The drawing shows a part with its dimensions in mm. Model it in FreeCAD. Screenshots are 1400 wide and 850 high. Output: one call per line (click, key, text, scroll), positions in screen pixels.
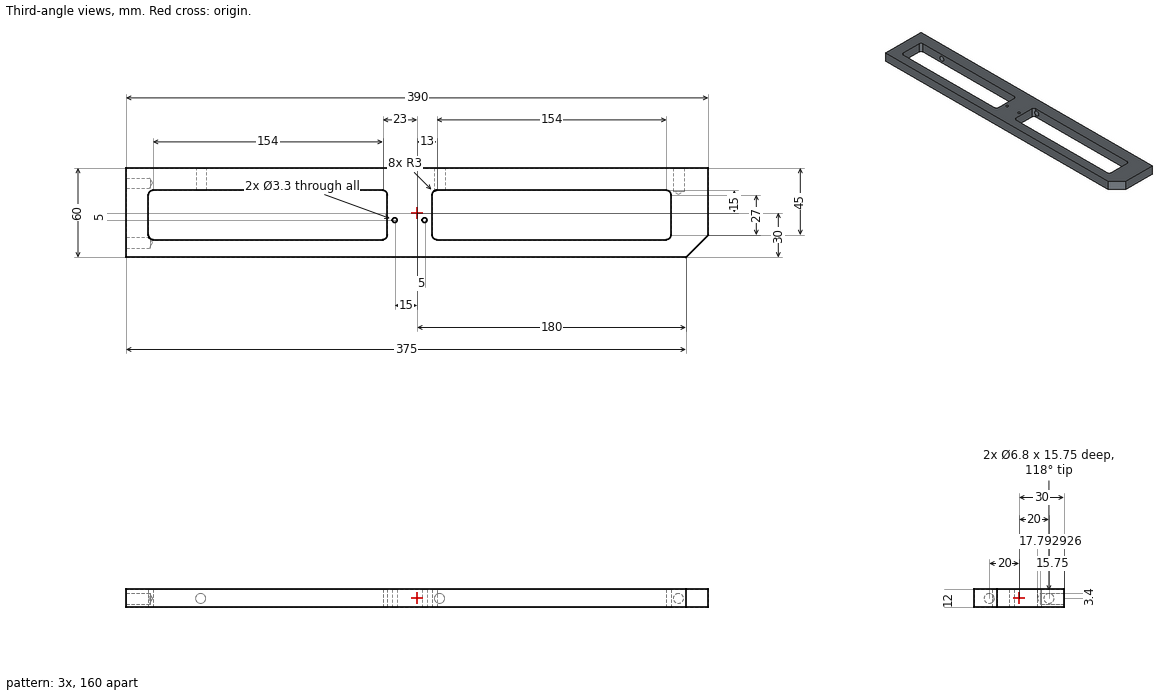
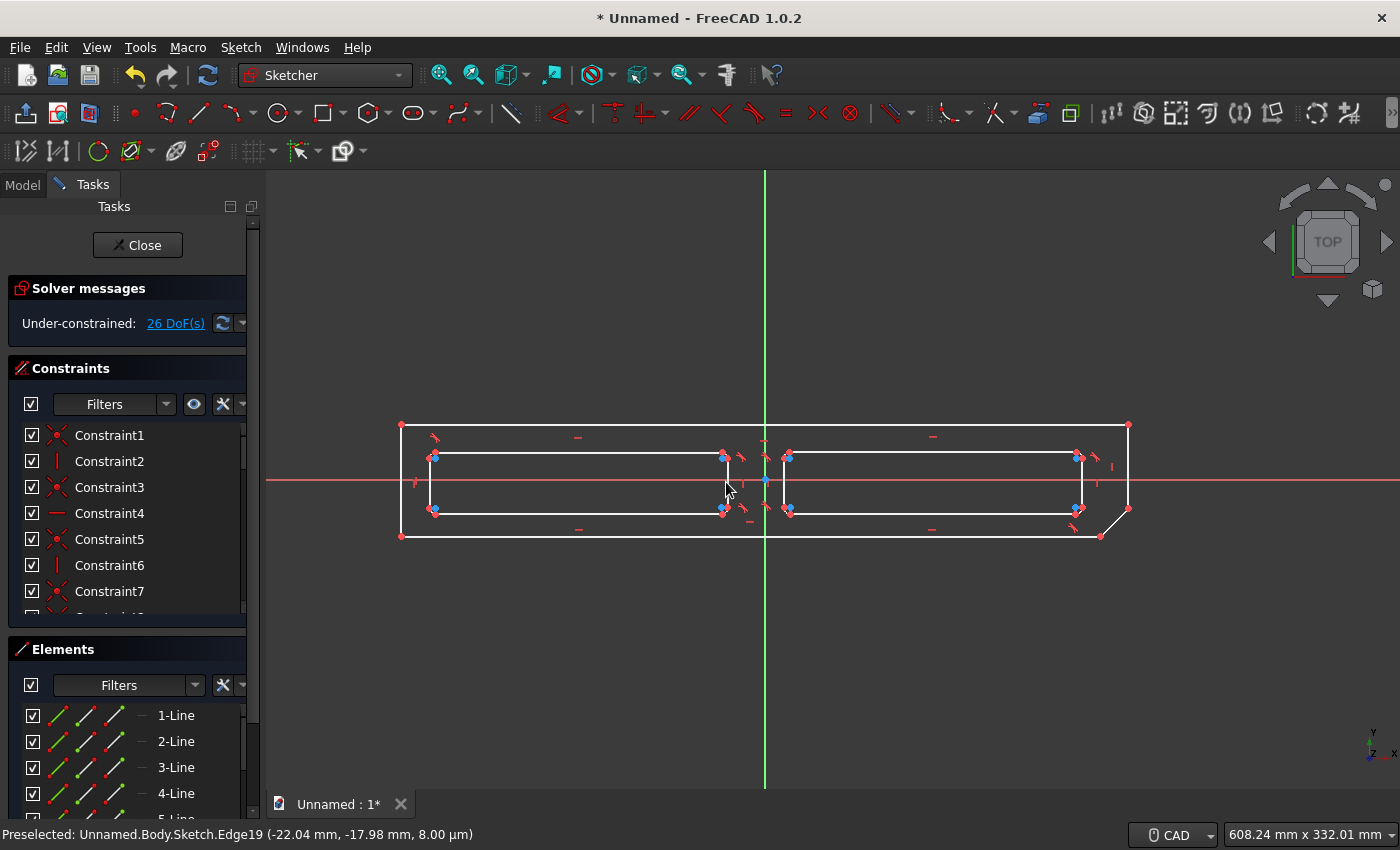
click(665, 514)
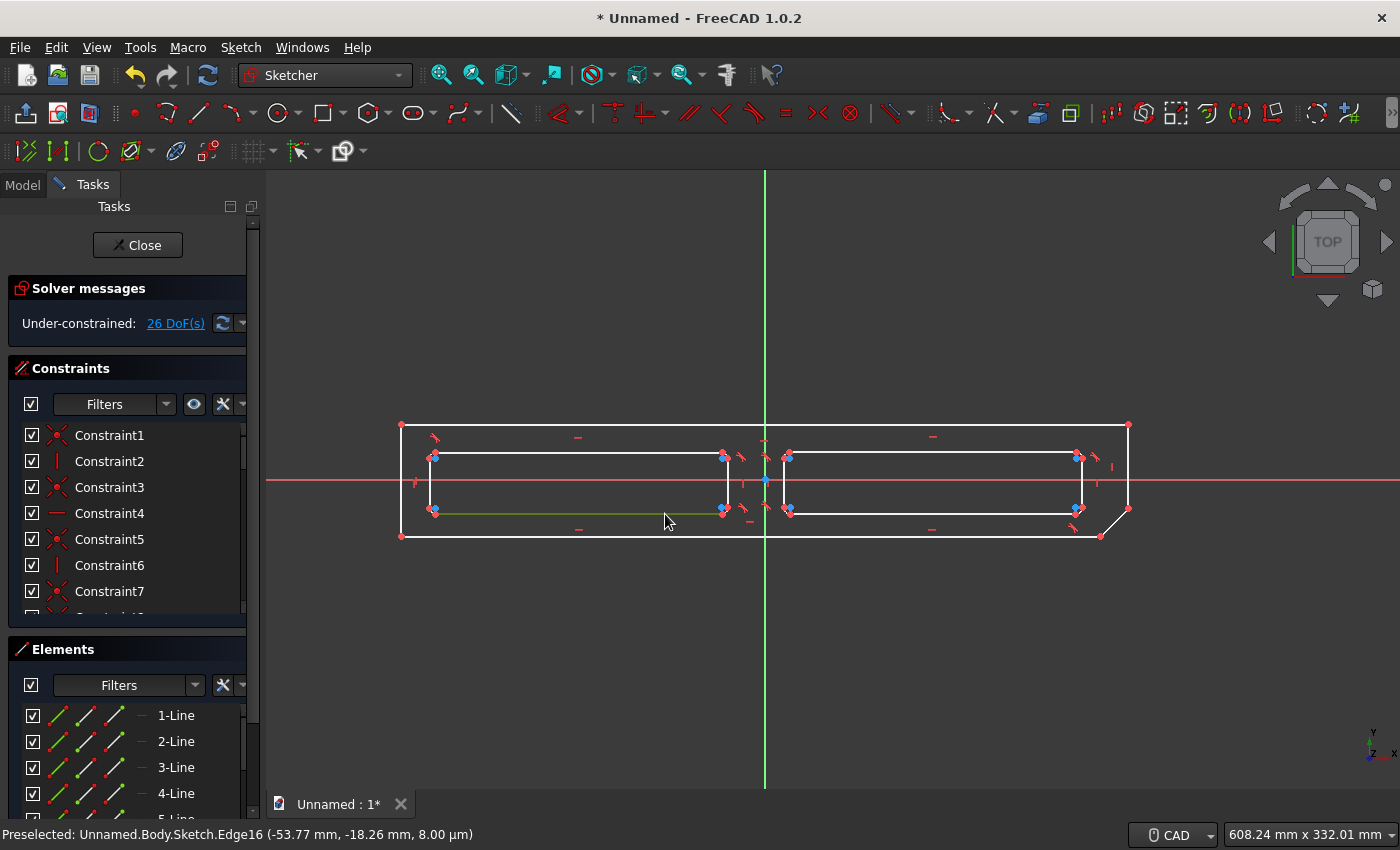
scroll(726, 512, up, 6)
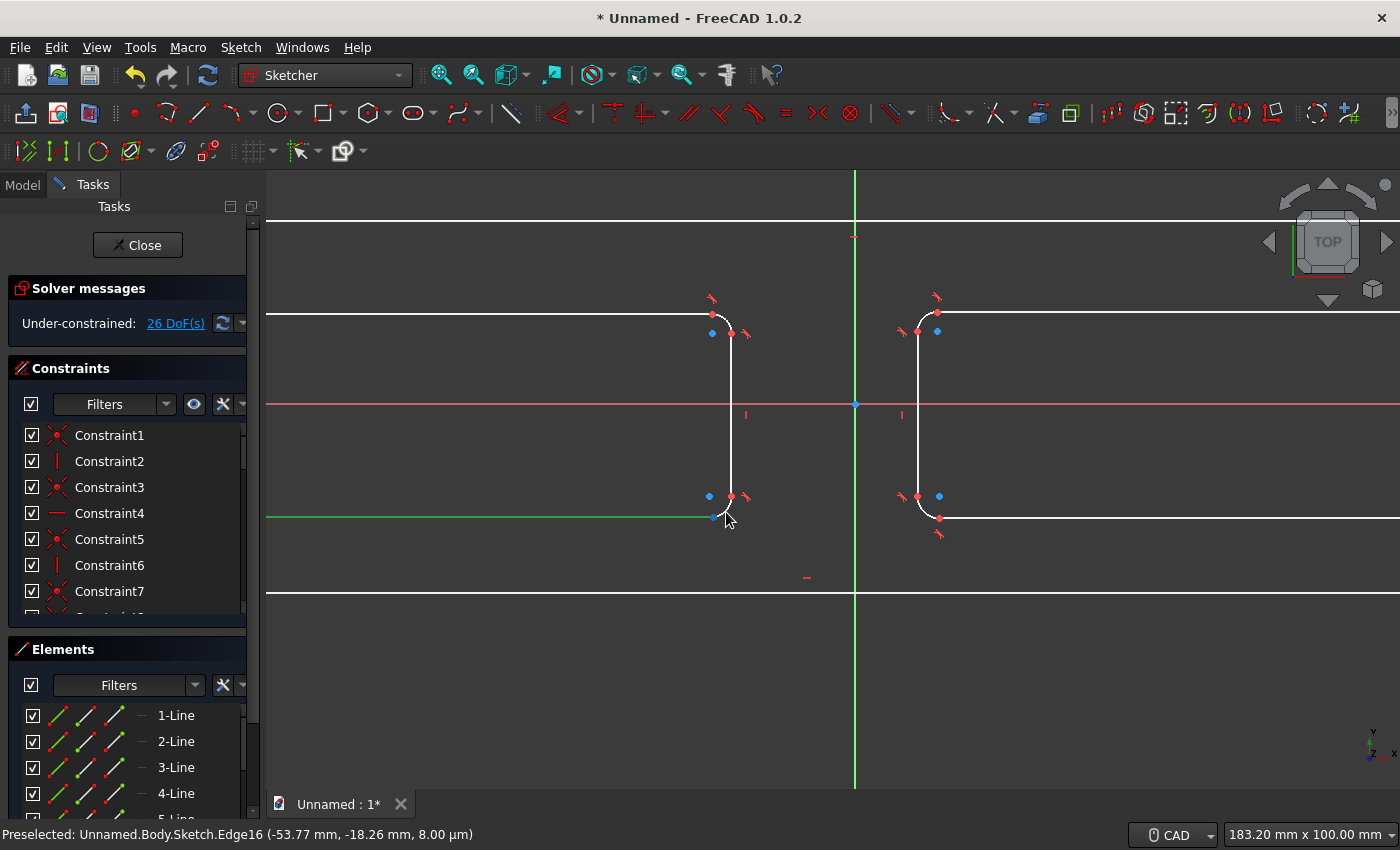
click(726, 510)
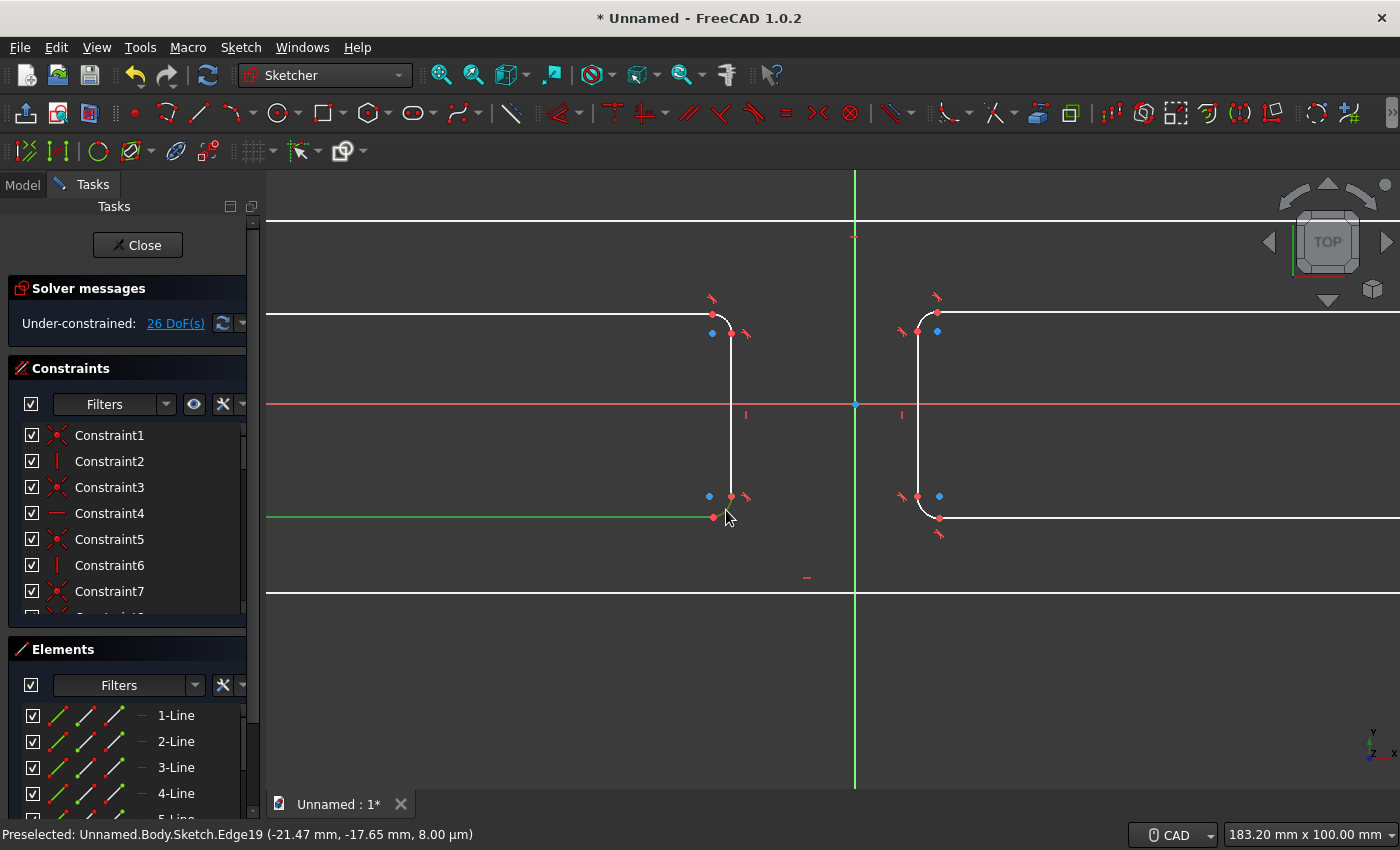
click(754, 114)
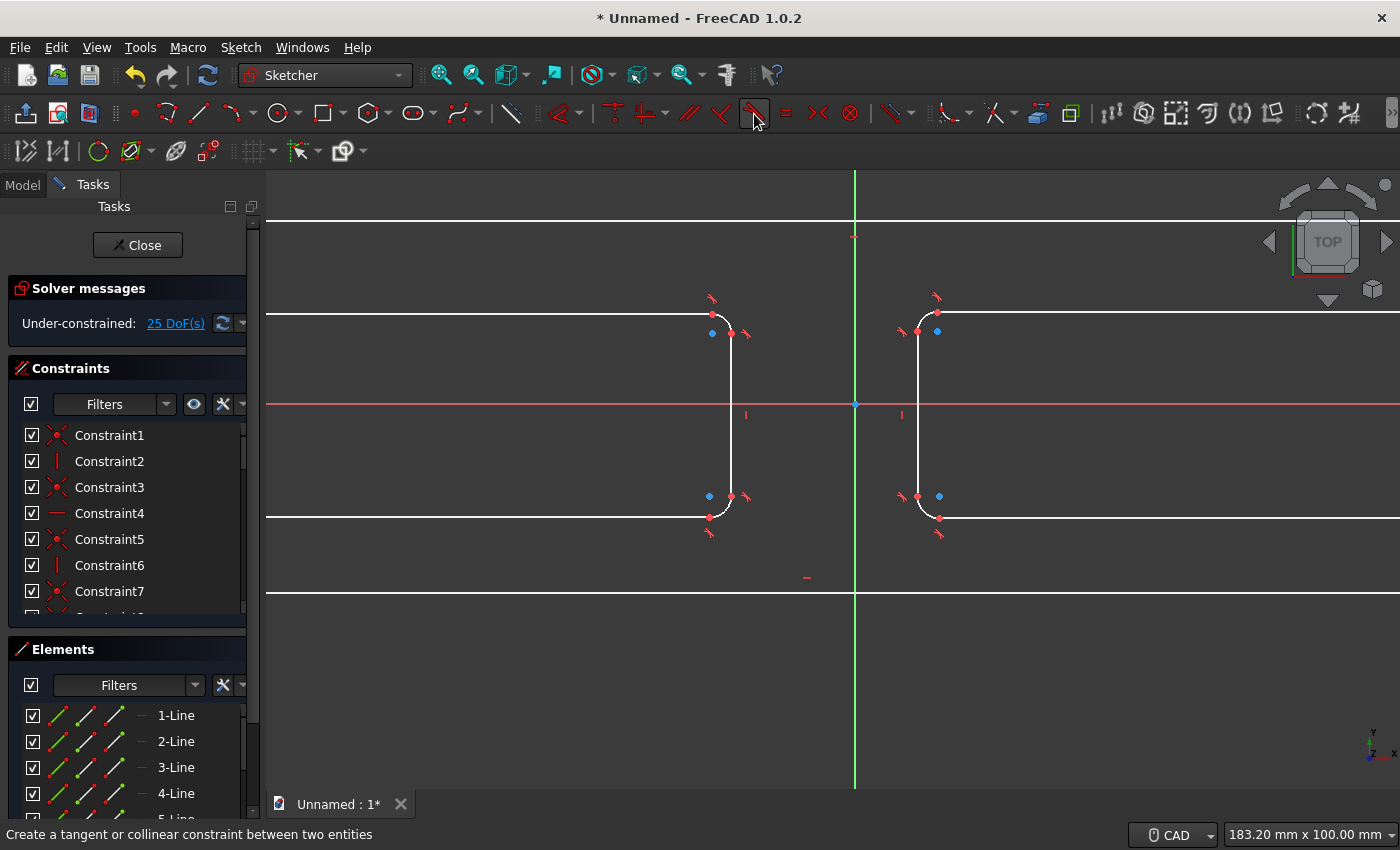
click(425, 517)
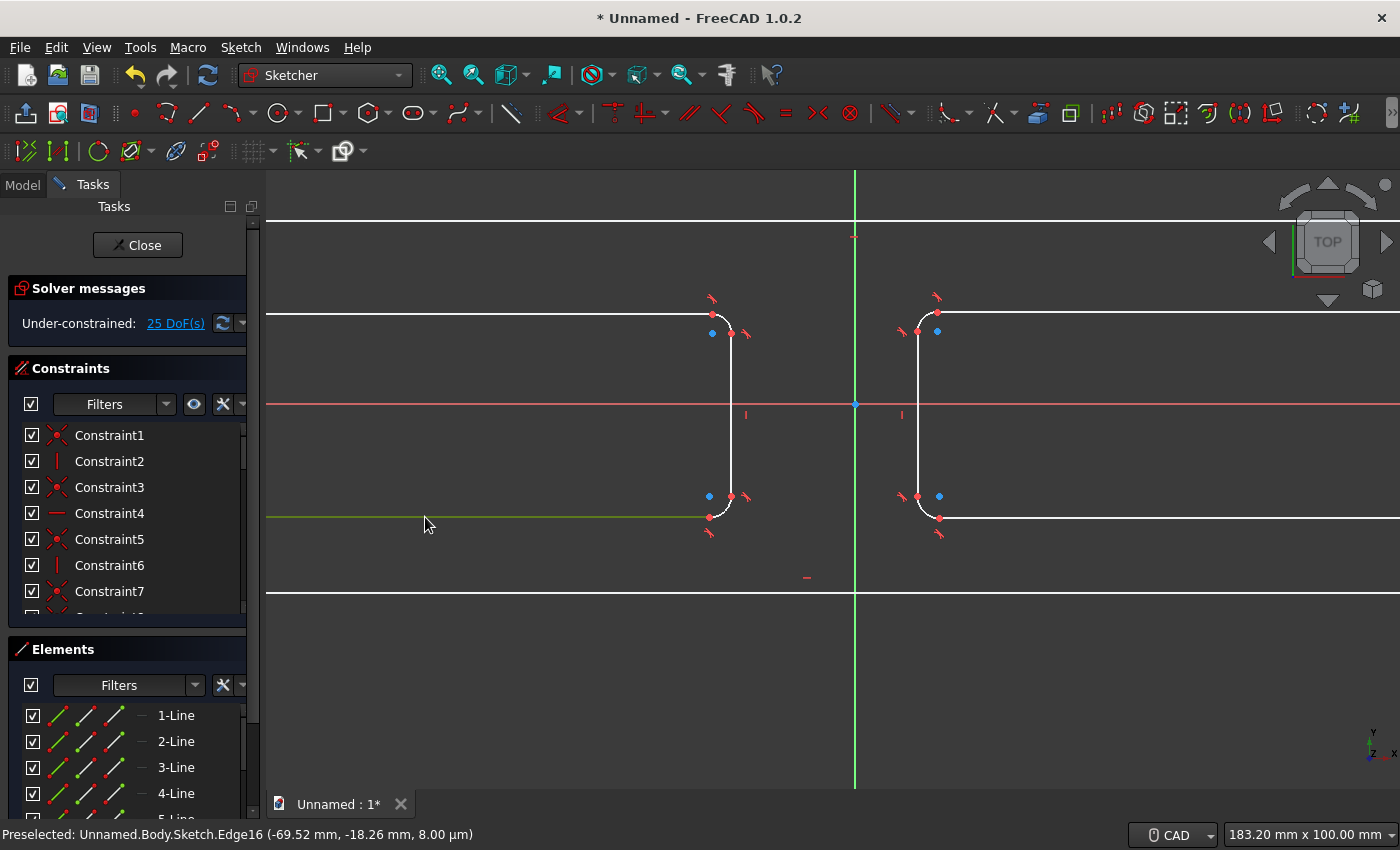
scroll(725, 512, down, 6)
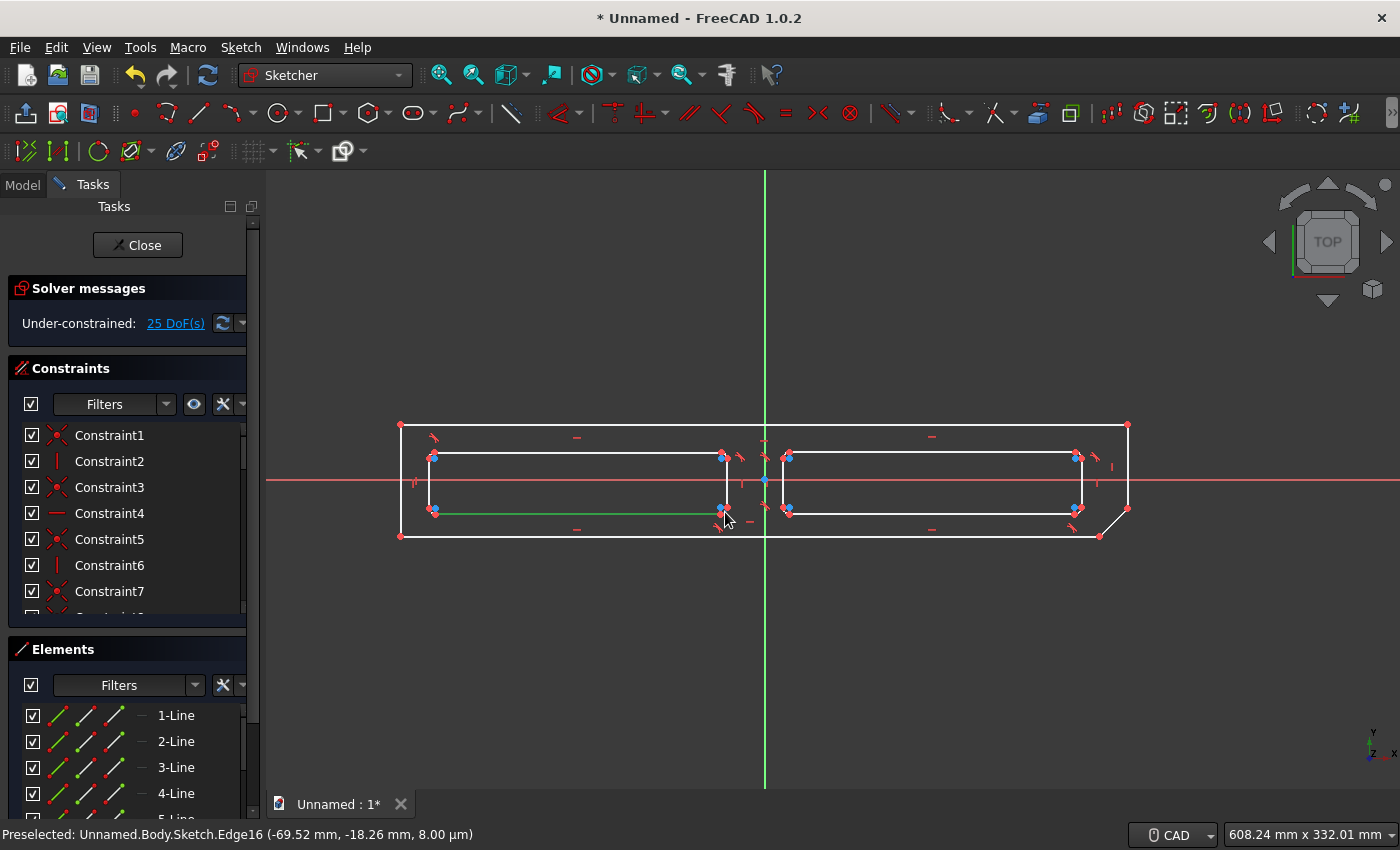
scroll(431, 512, up, 6)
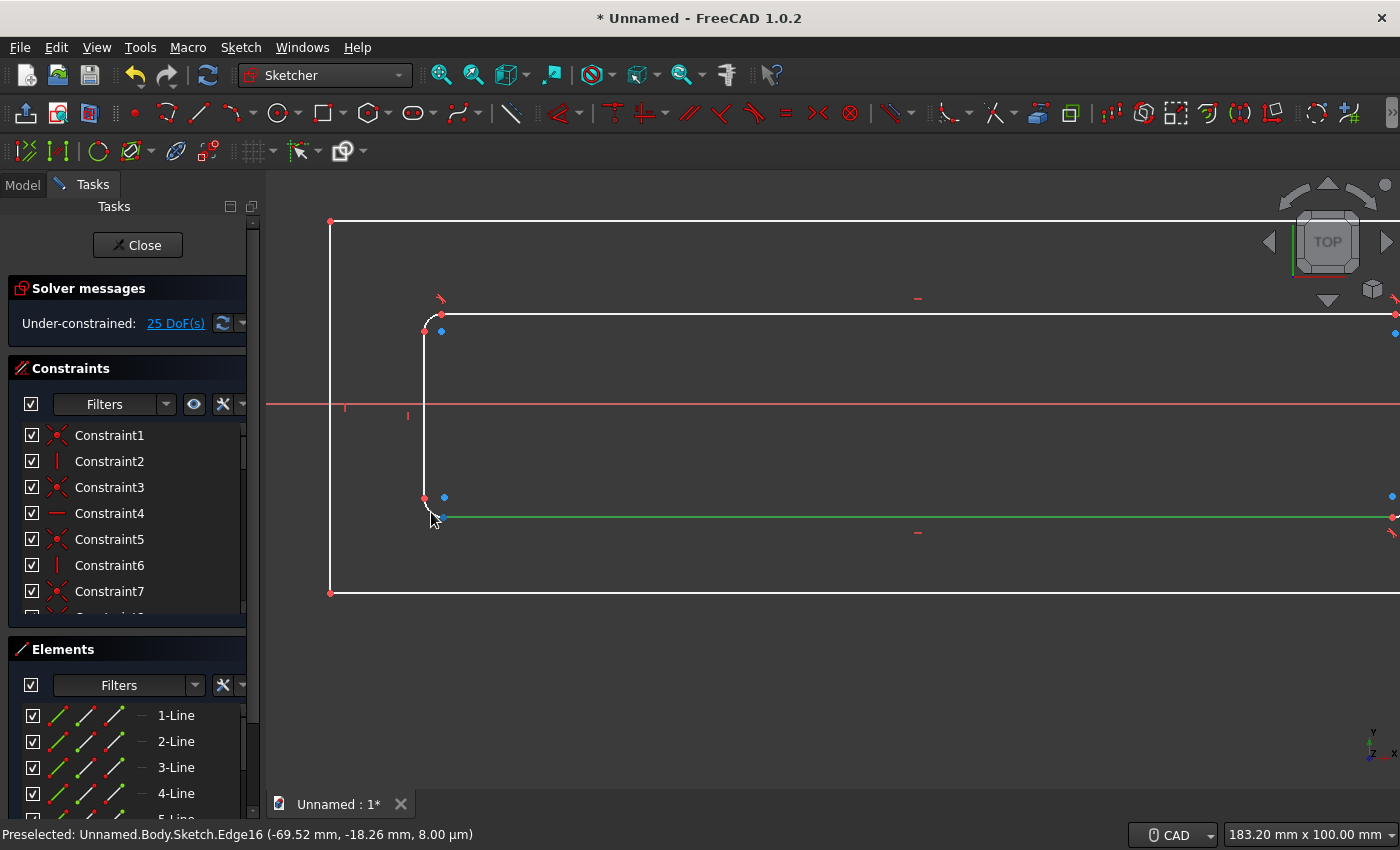
click(430, 512)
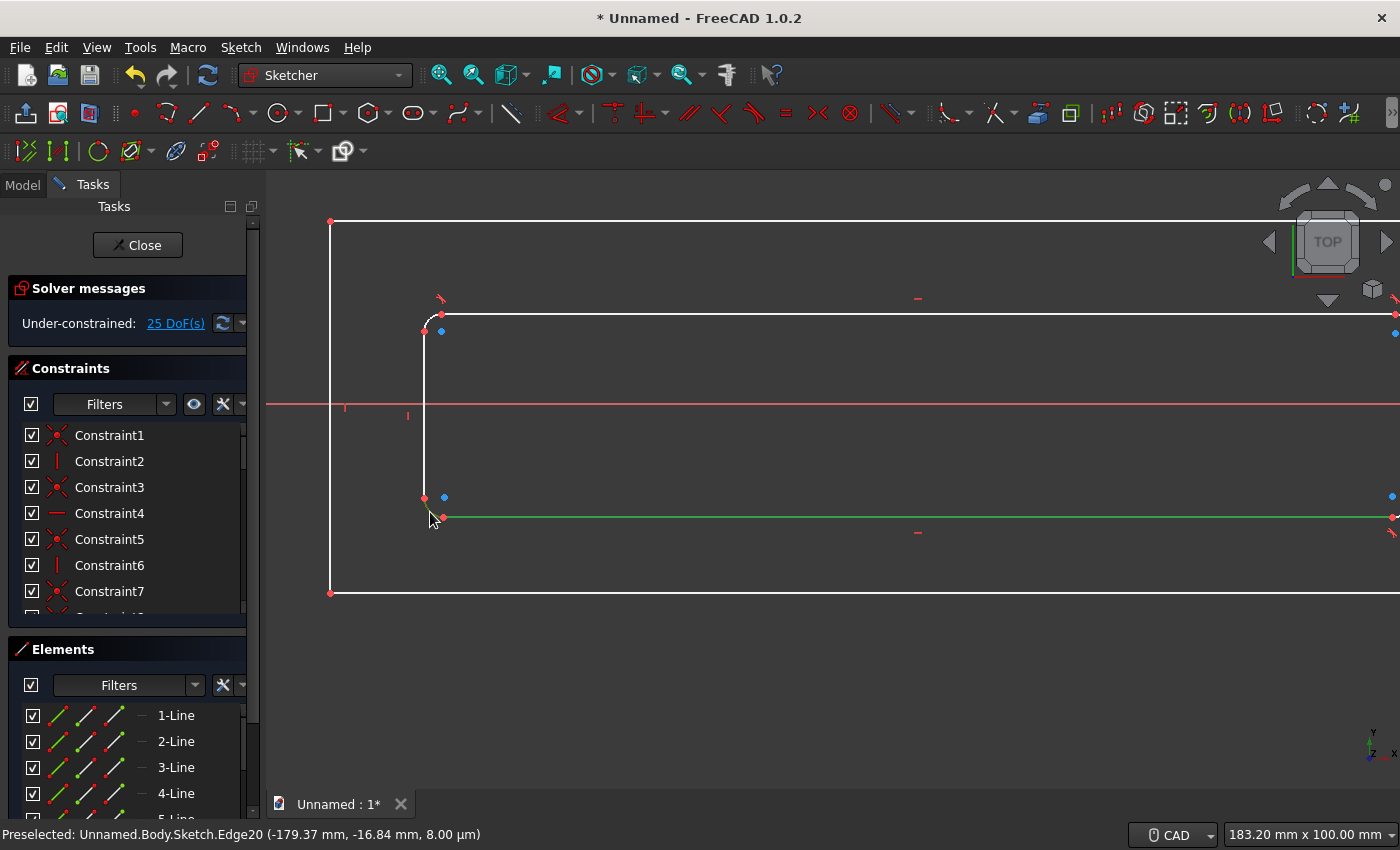
click(754, 114)